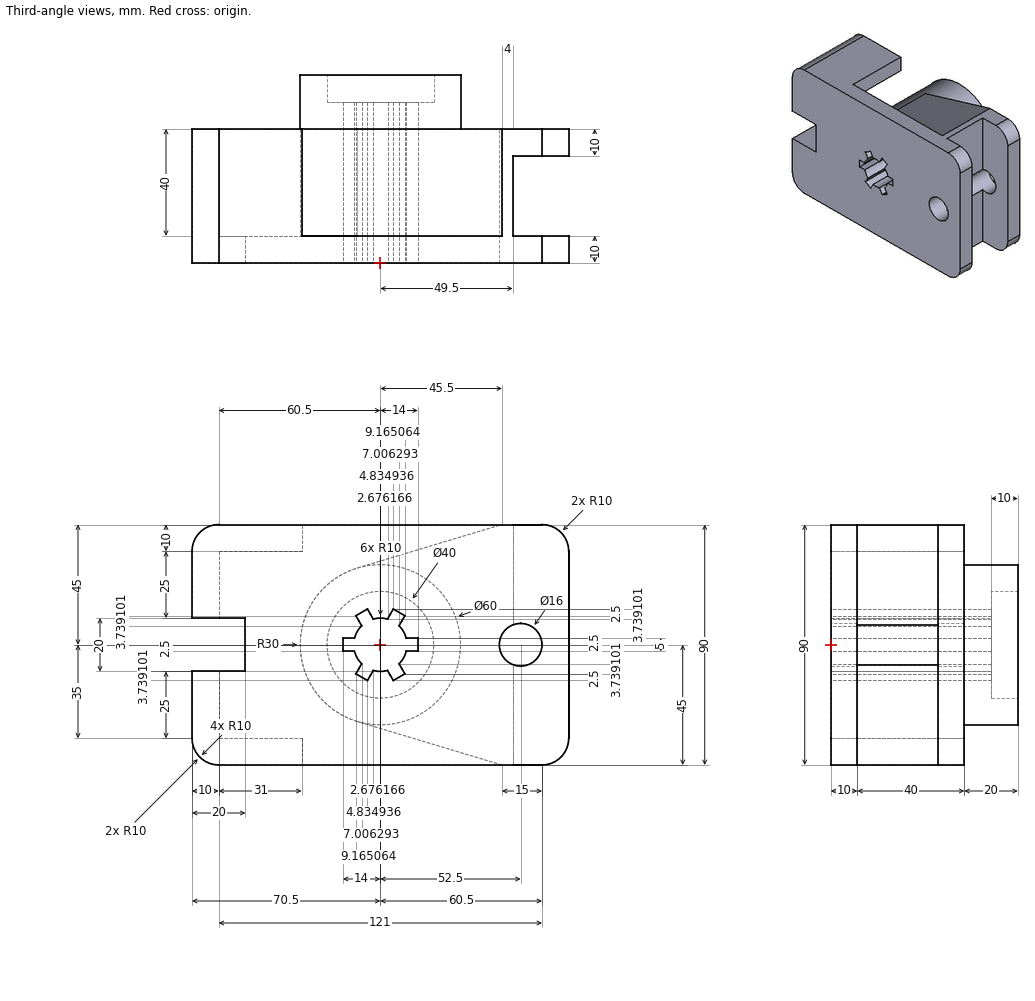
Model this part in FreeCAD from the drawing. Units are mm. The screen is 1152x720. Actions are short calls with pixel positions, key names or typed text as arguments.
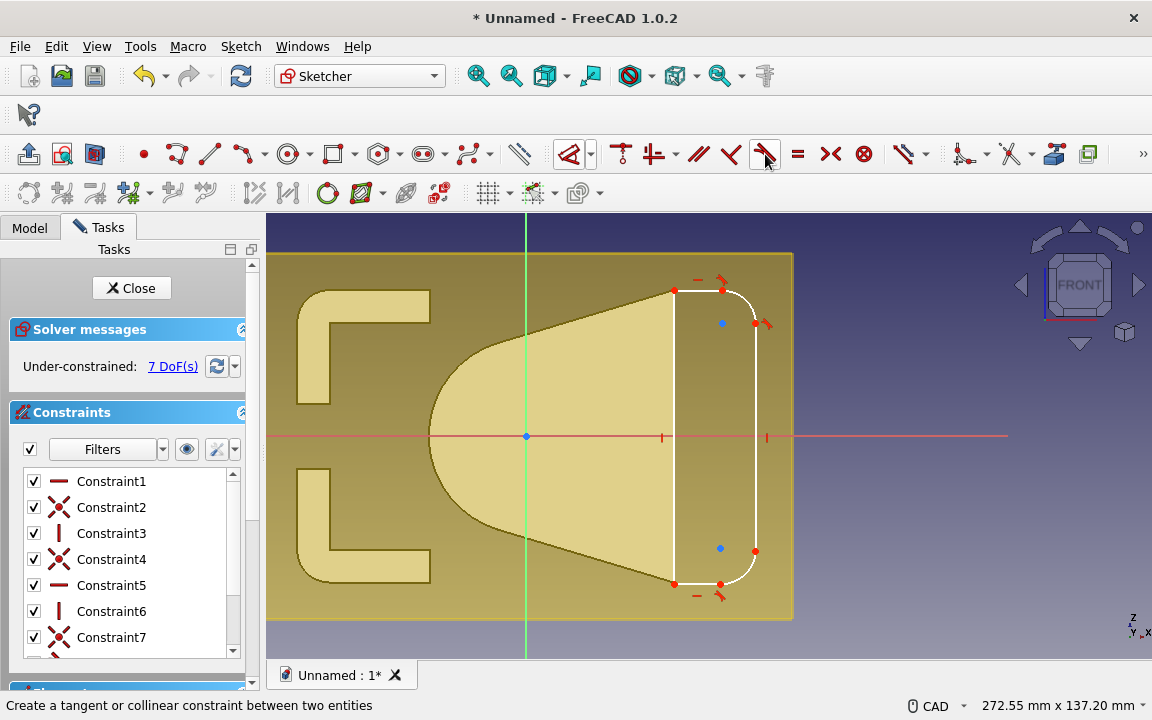
click(756, 392)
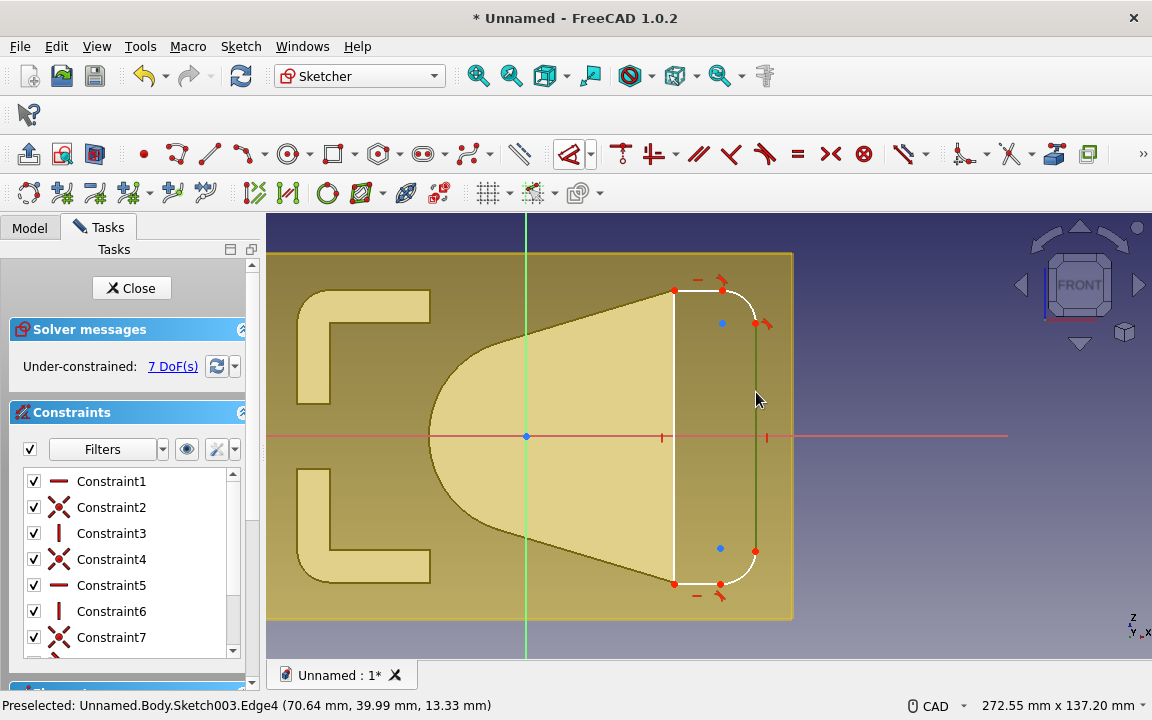
click(736, 581)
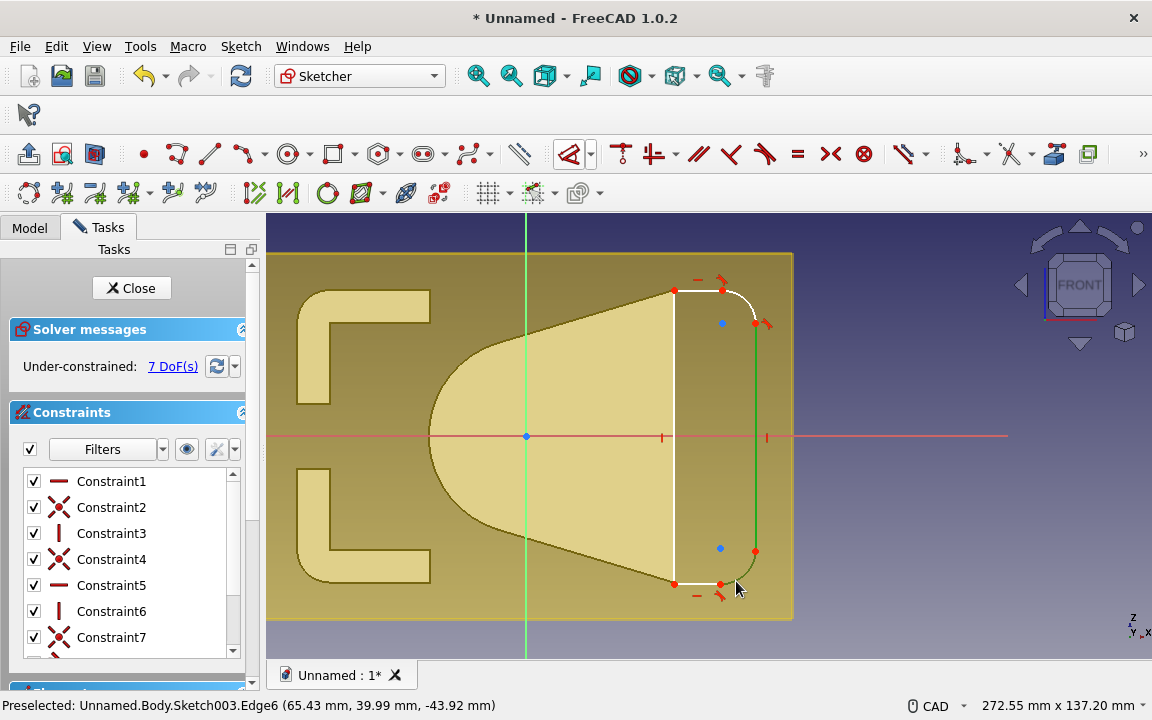
click(765, 154)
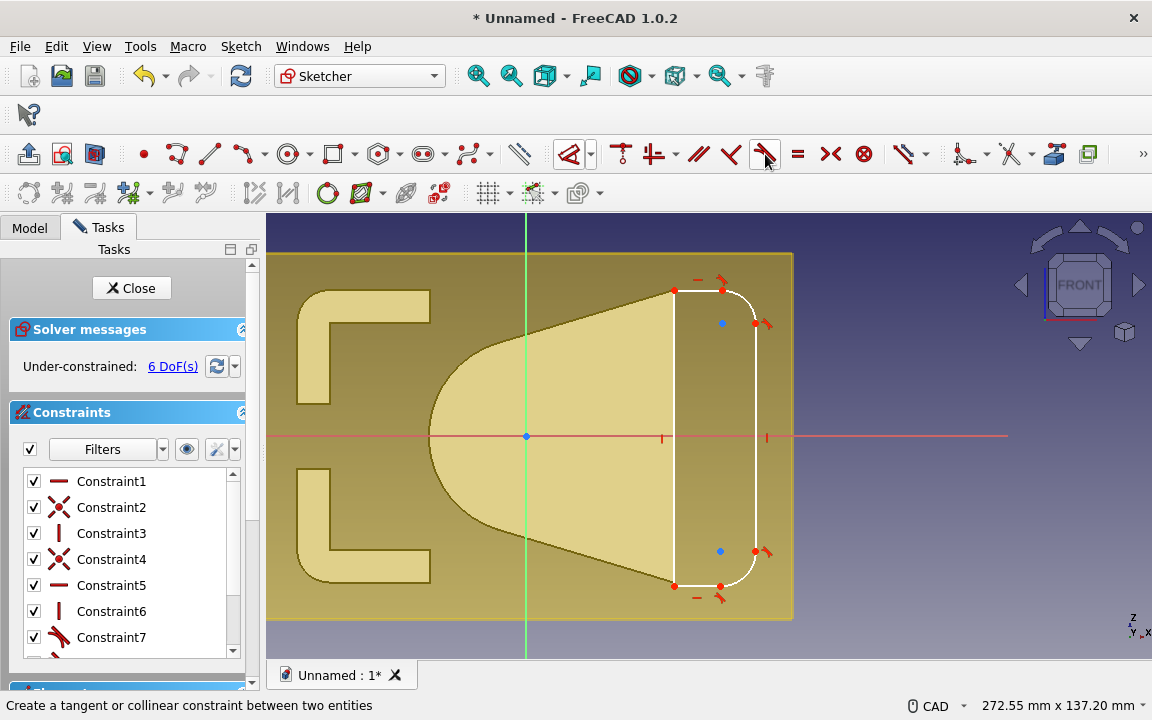
click(752, 309)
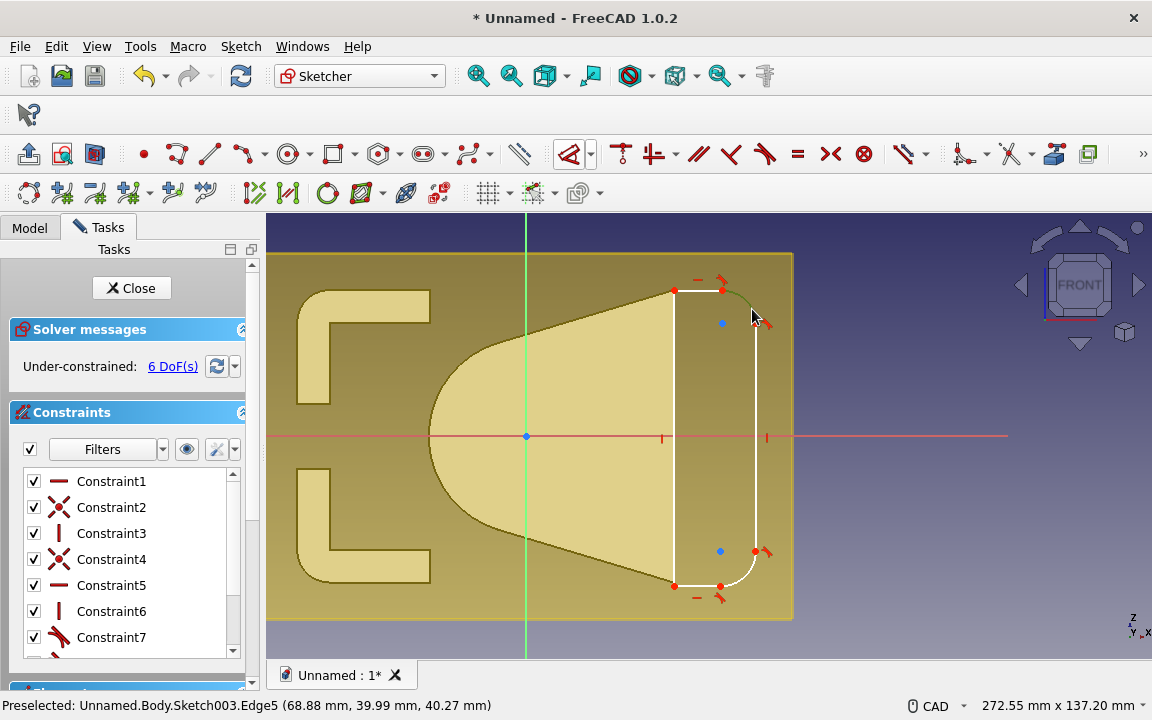
click(737, 582)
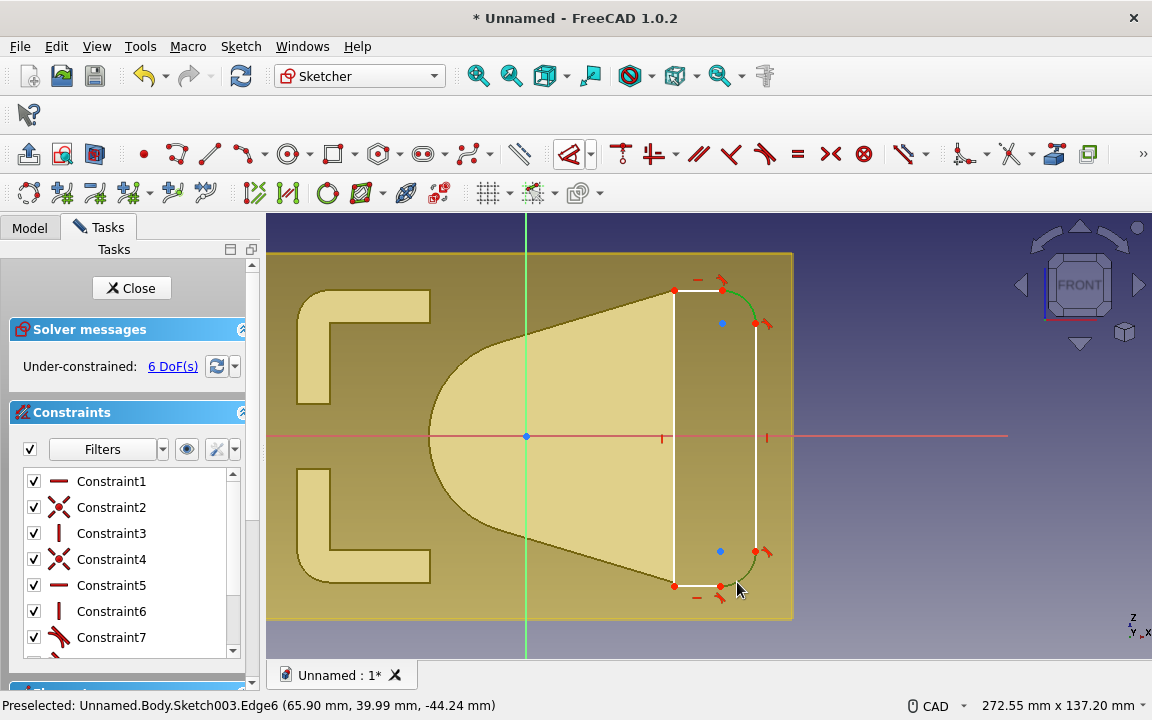
click(798, 154)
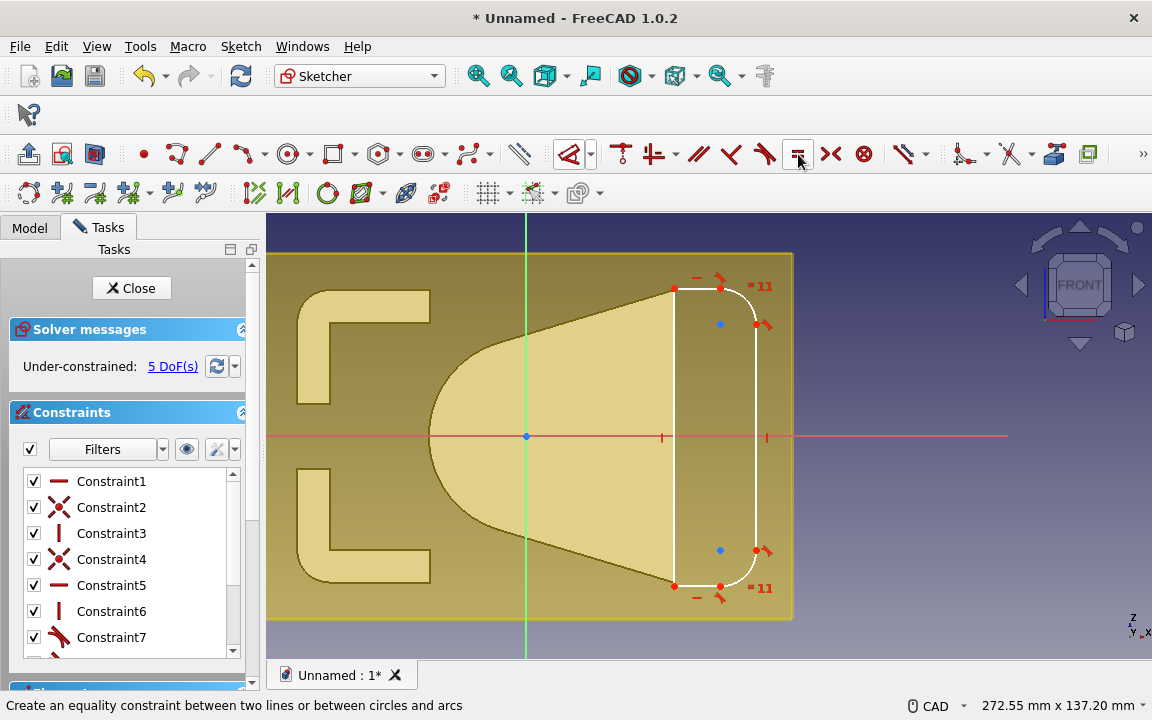
click(752, 308)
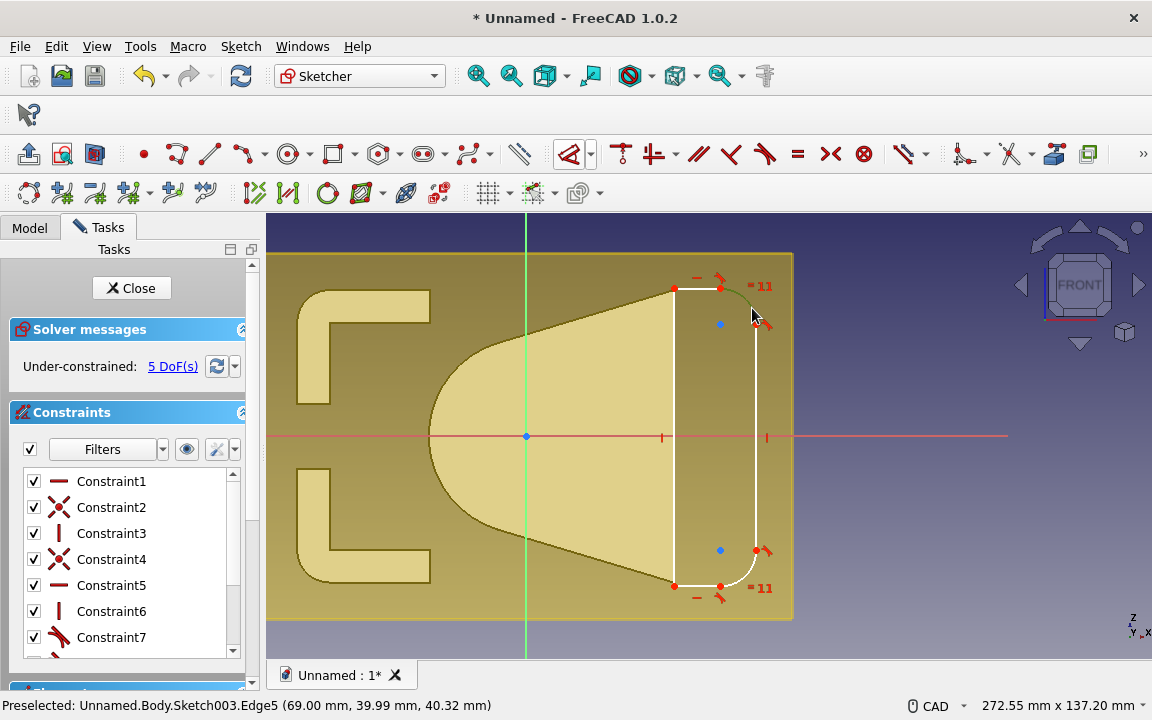
click(590, 154)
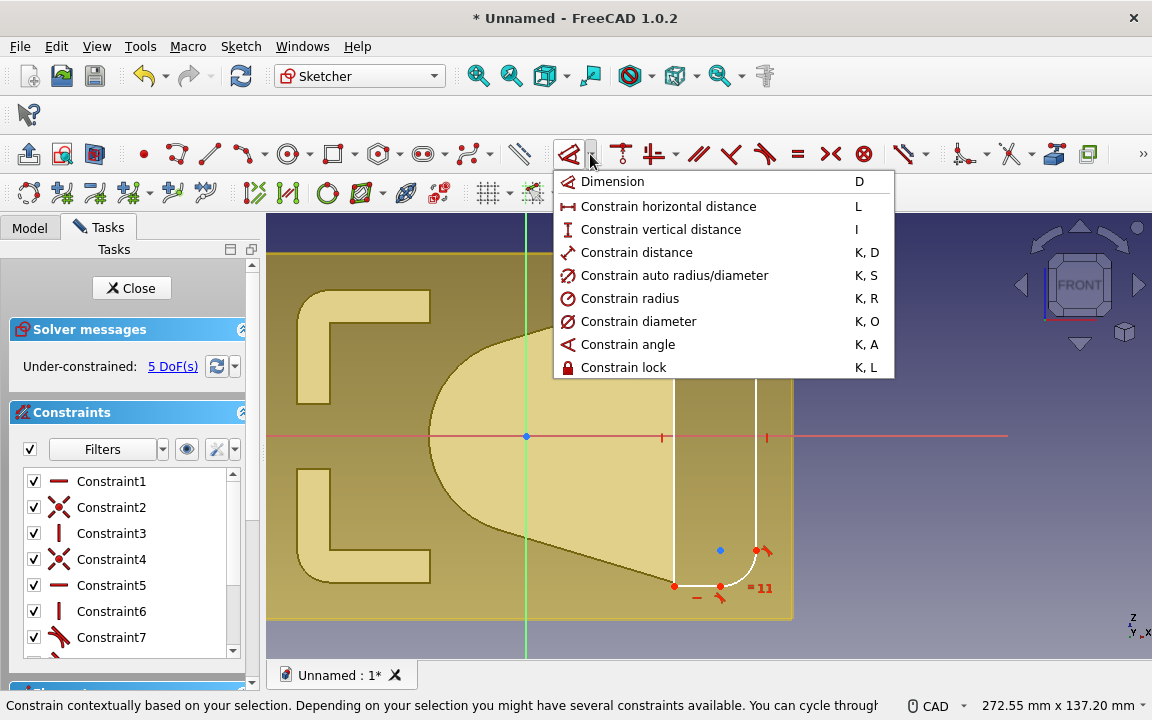
click(724, 298)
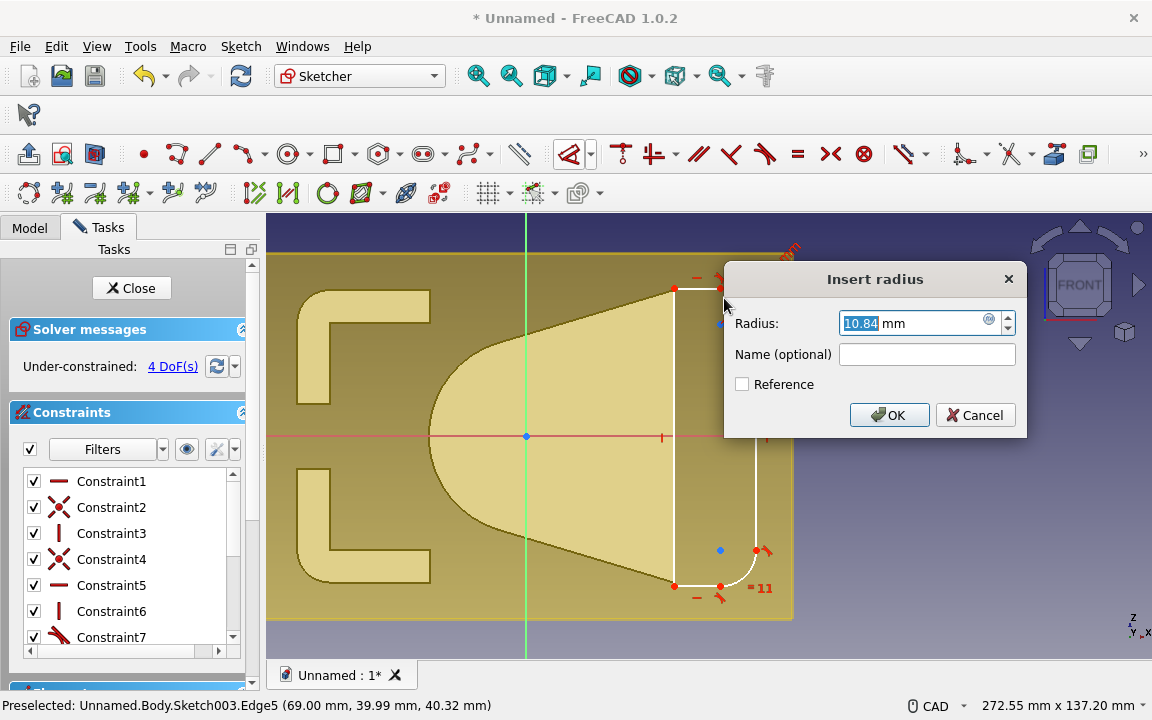
text(10)
key(Return)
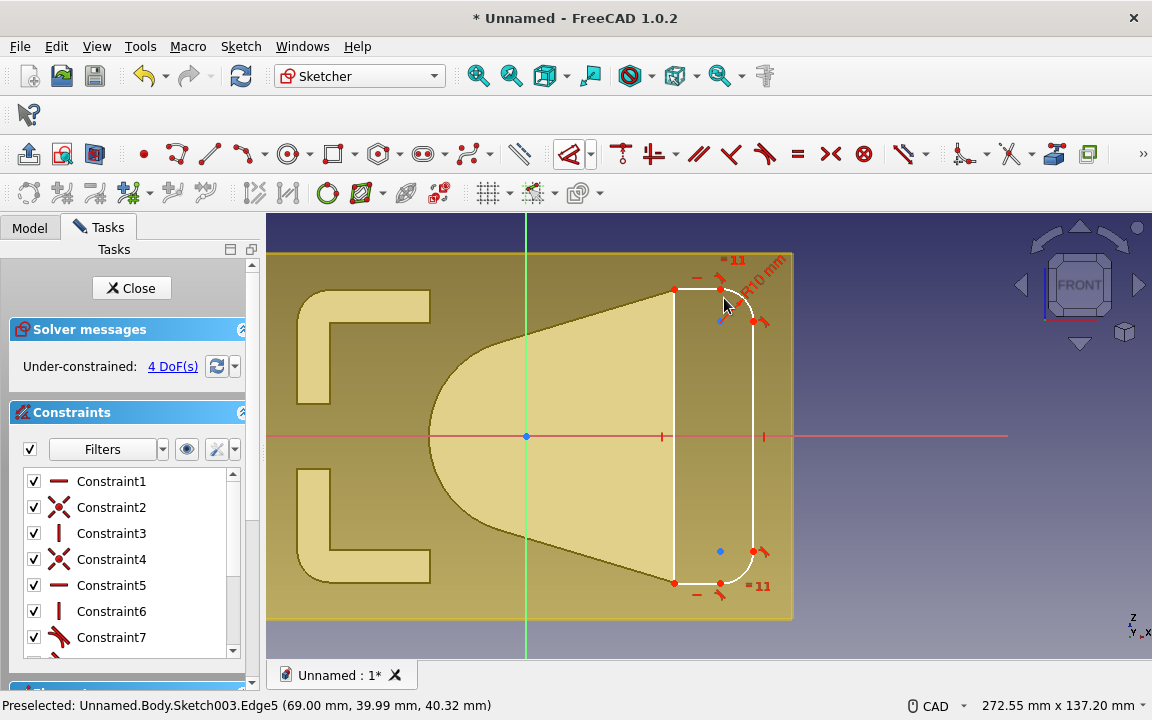
click(707, 584)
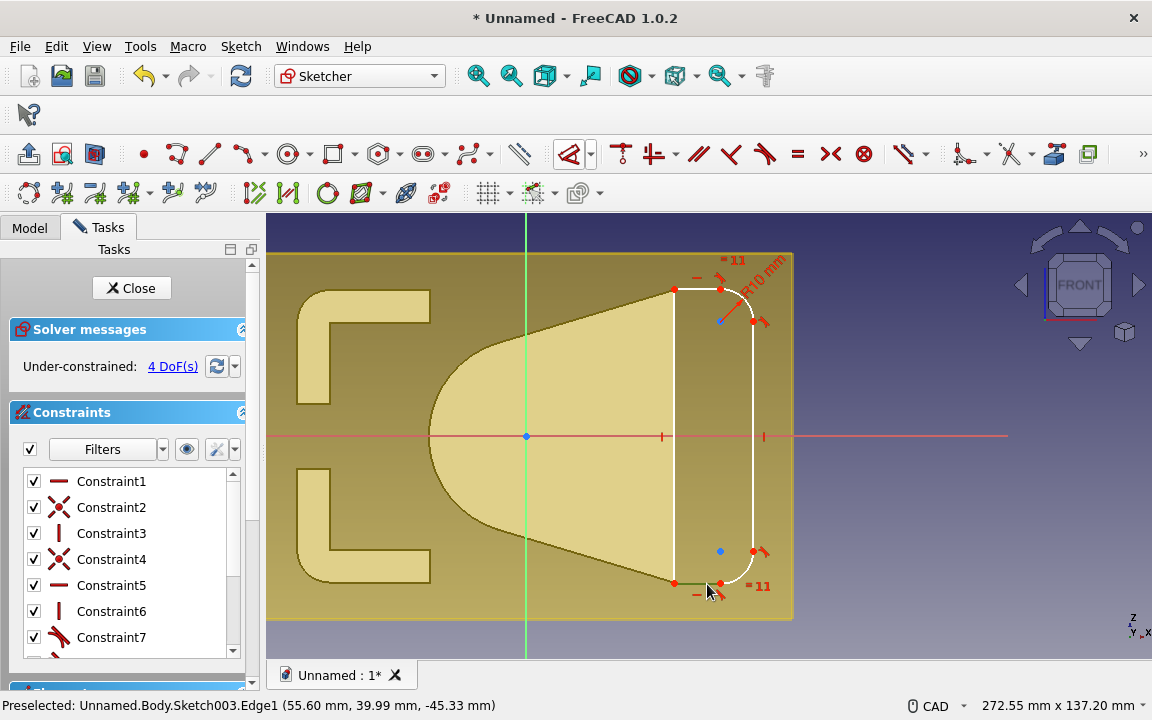
click(590, 154)